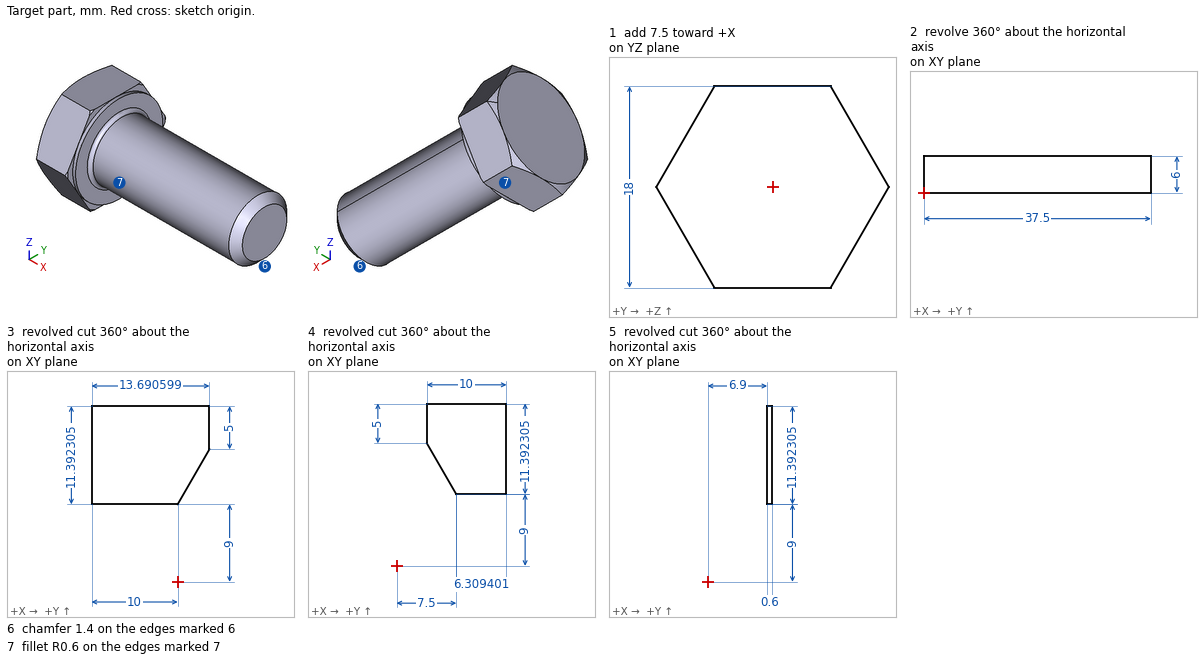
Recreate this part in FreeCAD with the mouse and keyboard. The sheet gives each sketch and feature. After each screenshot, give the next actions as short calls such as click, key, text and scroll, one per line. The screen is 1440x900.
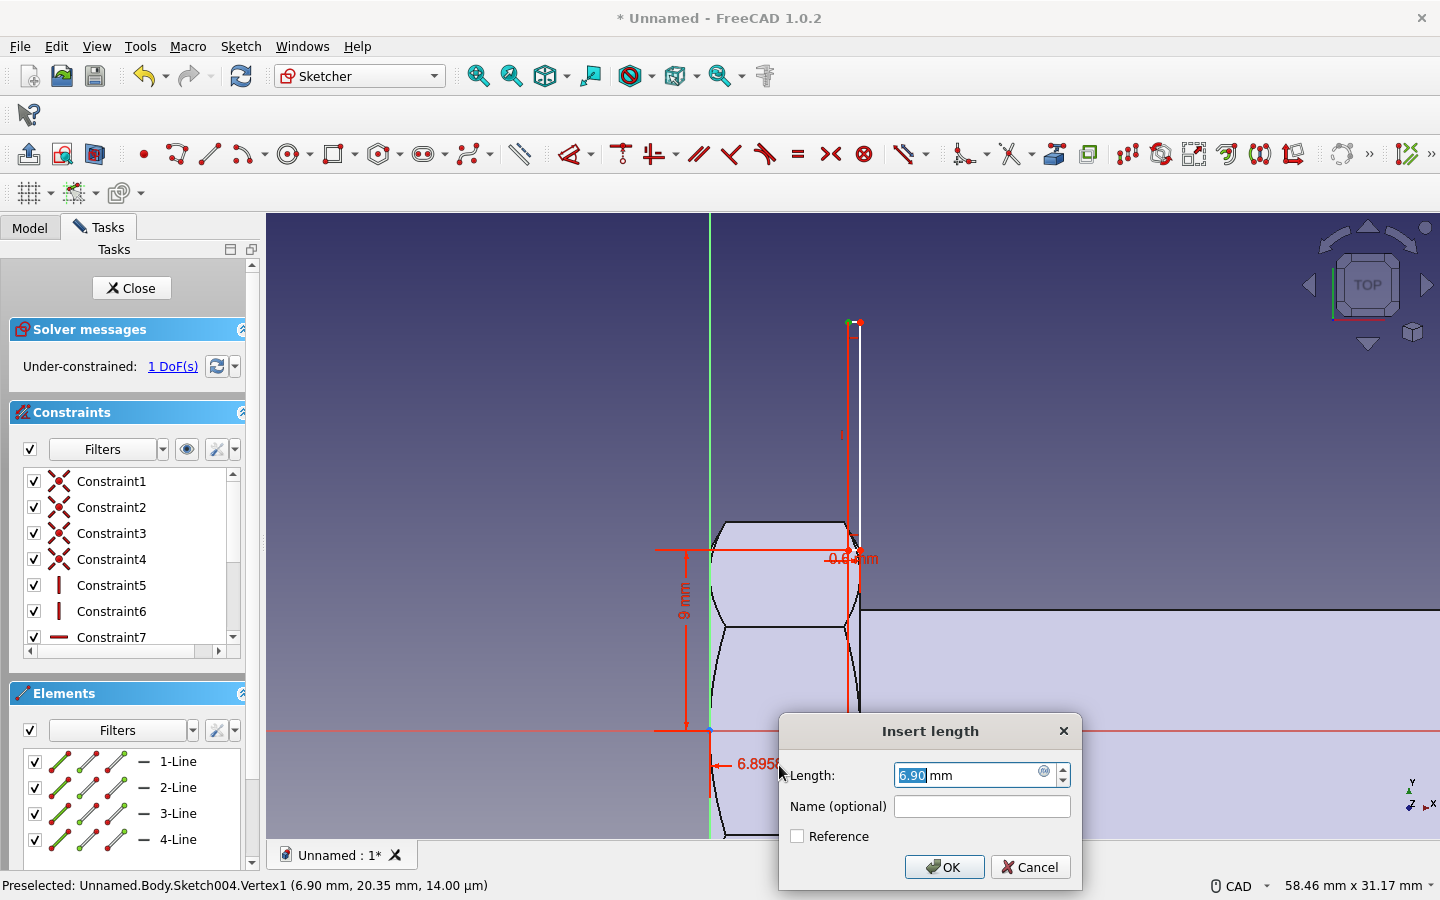
text(6.9)
key(Return)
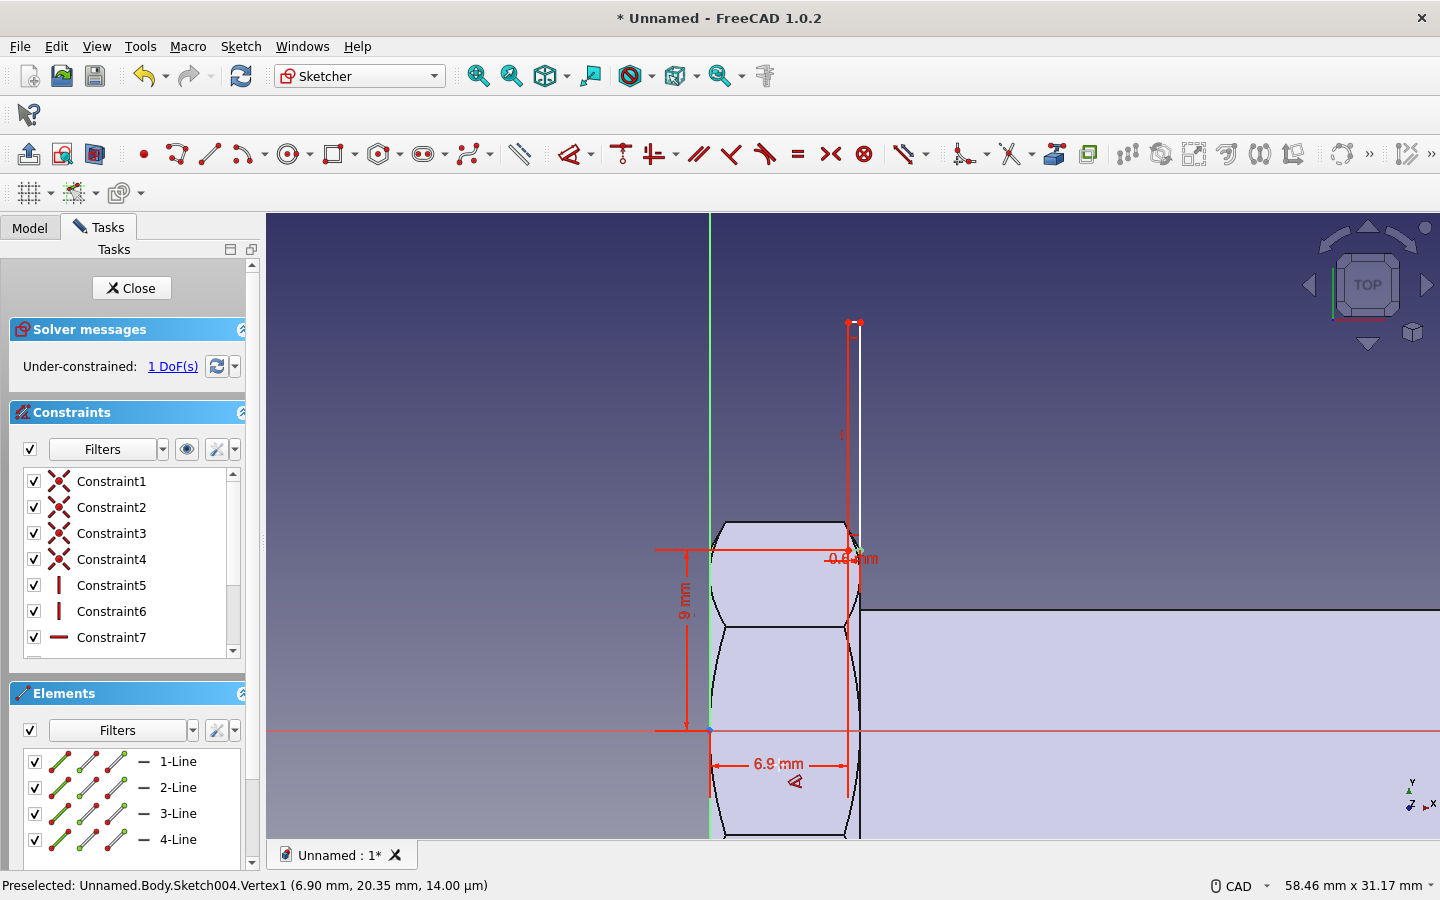
click(848, 391)
click(882, 436)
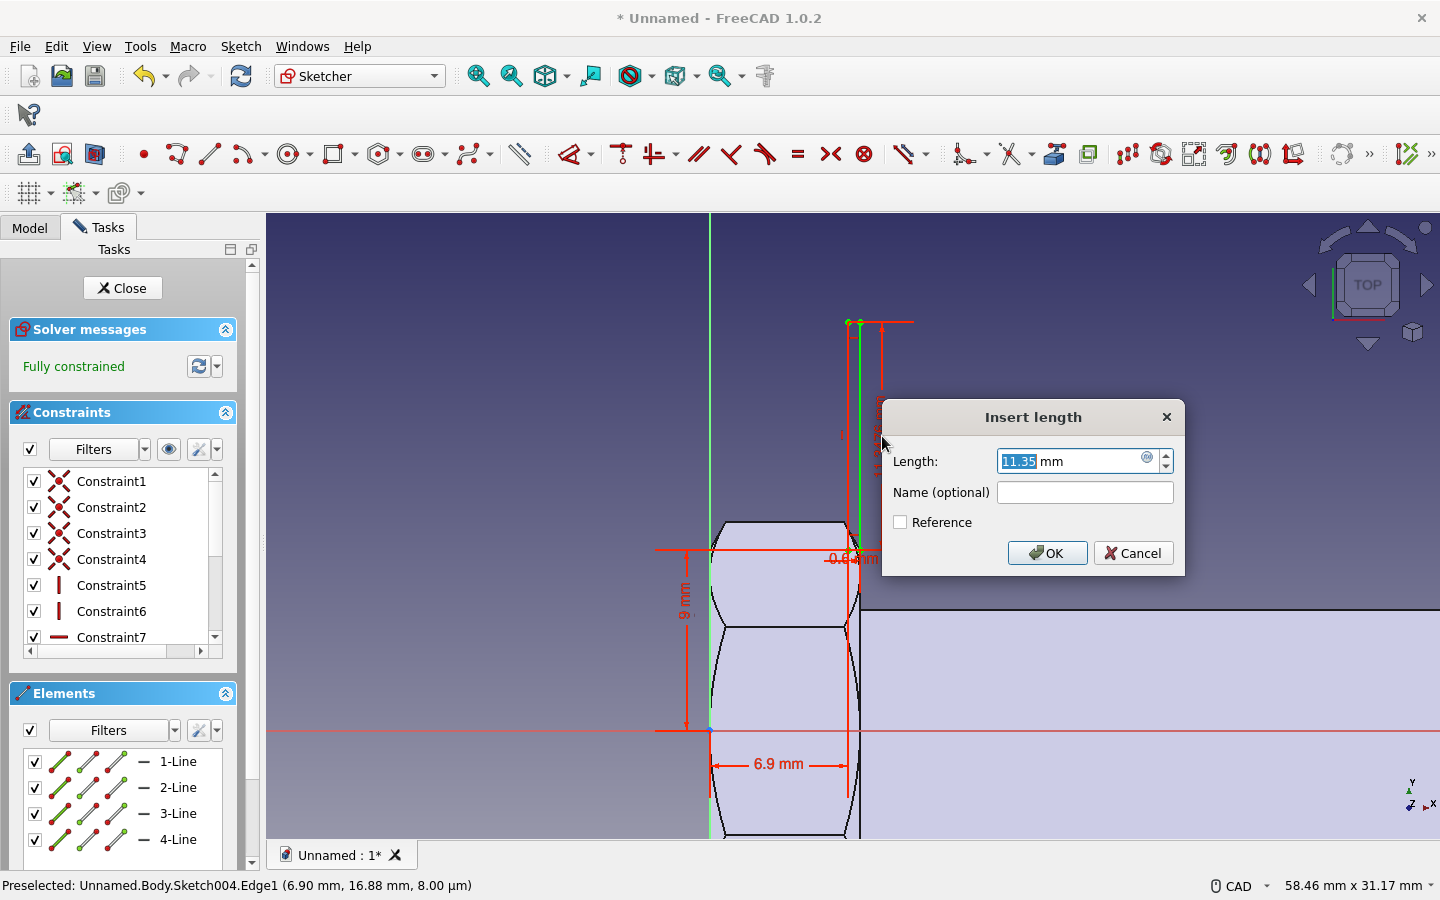
text(11.392305)
key(Return)
key(Escape)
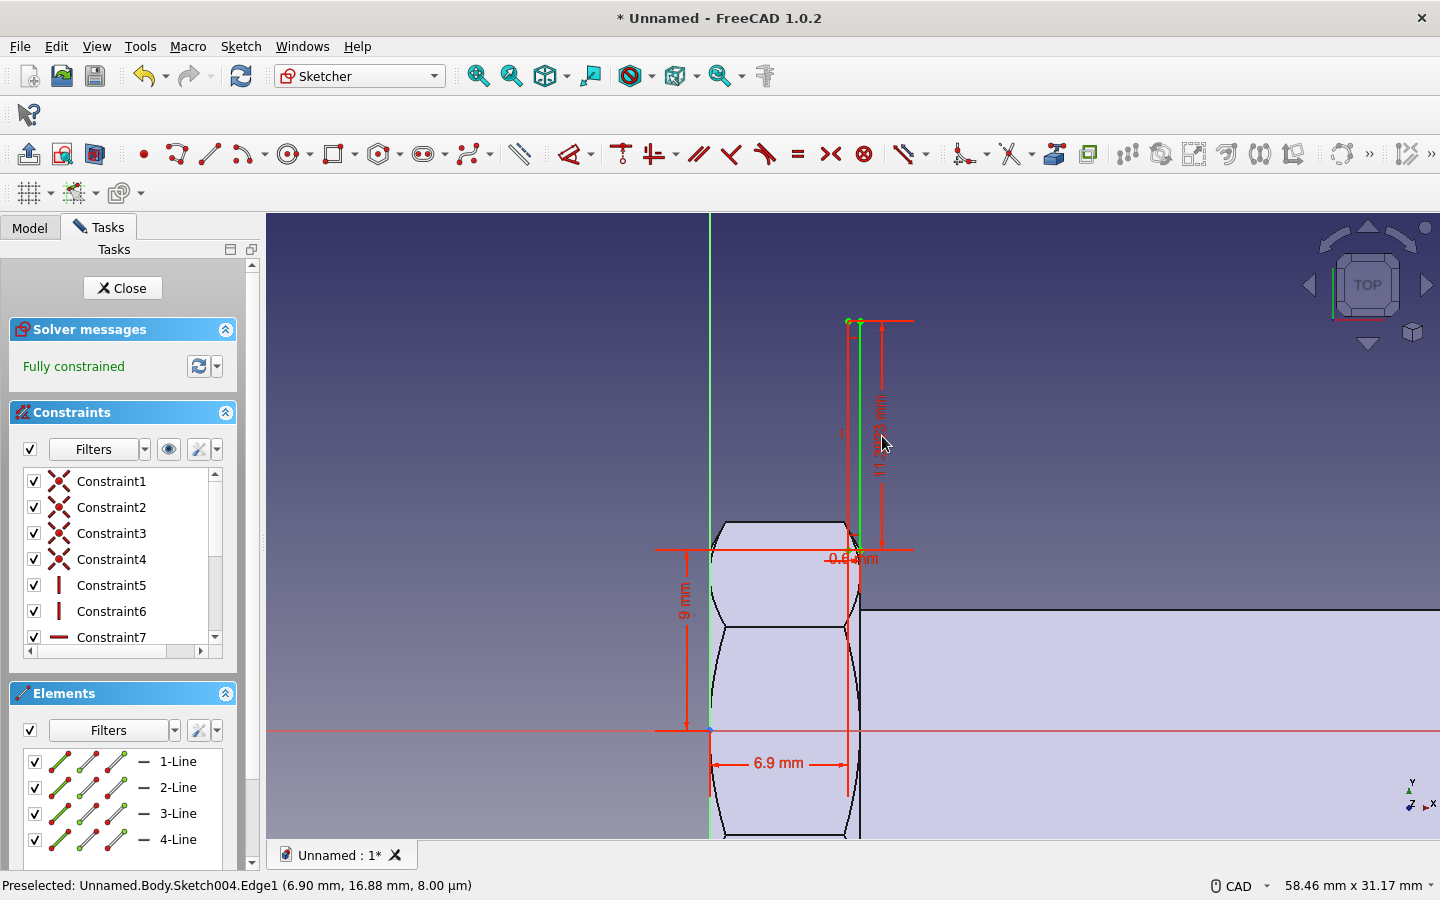
click(123, 288)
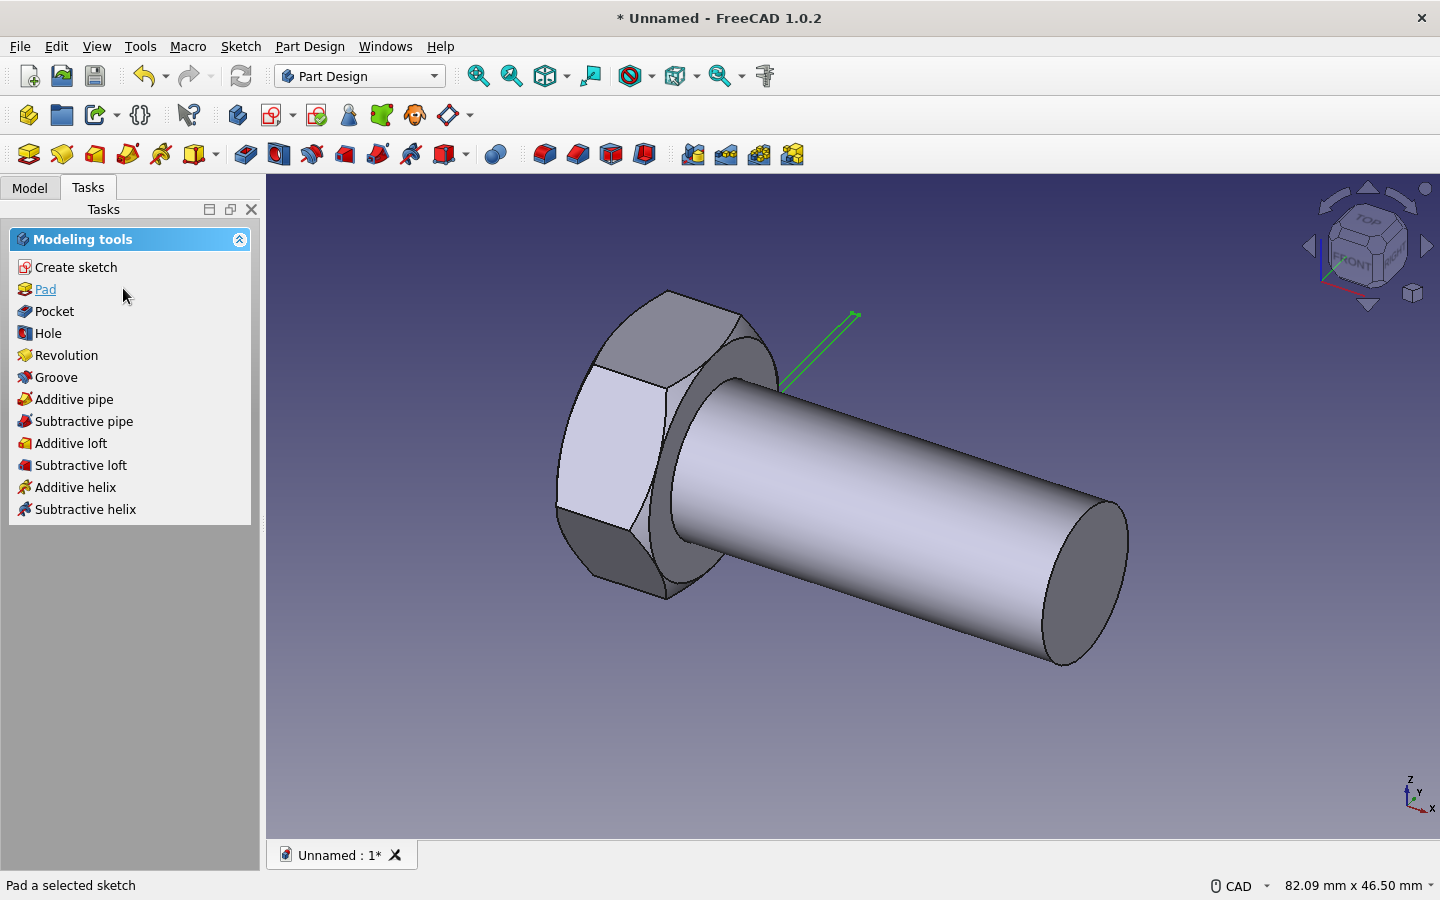
click(312, 154)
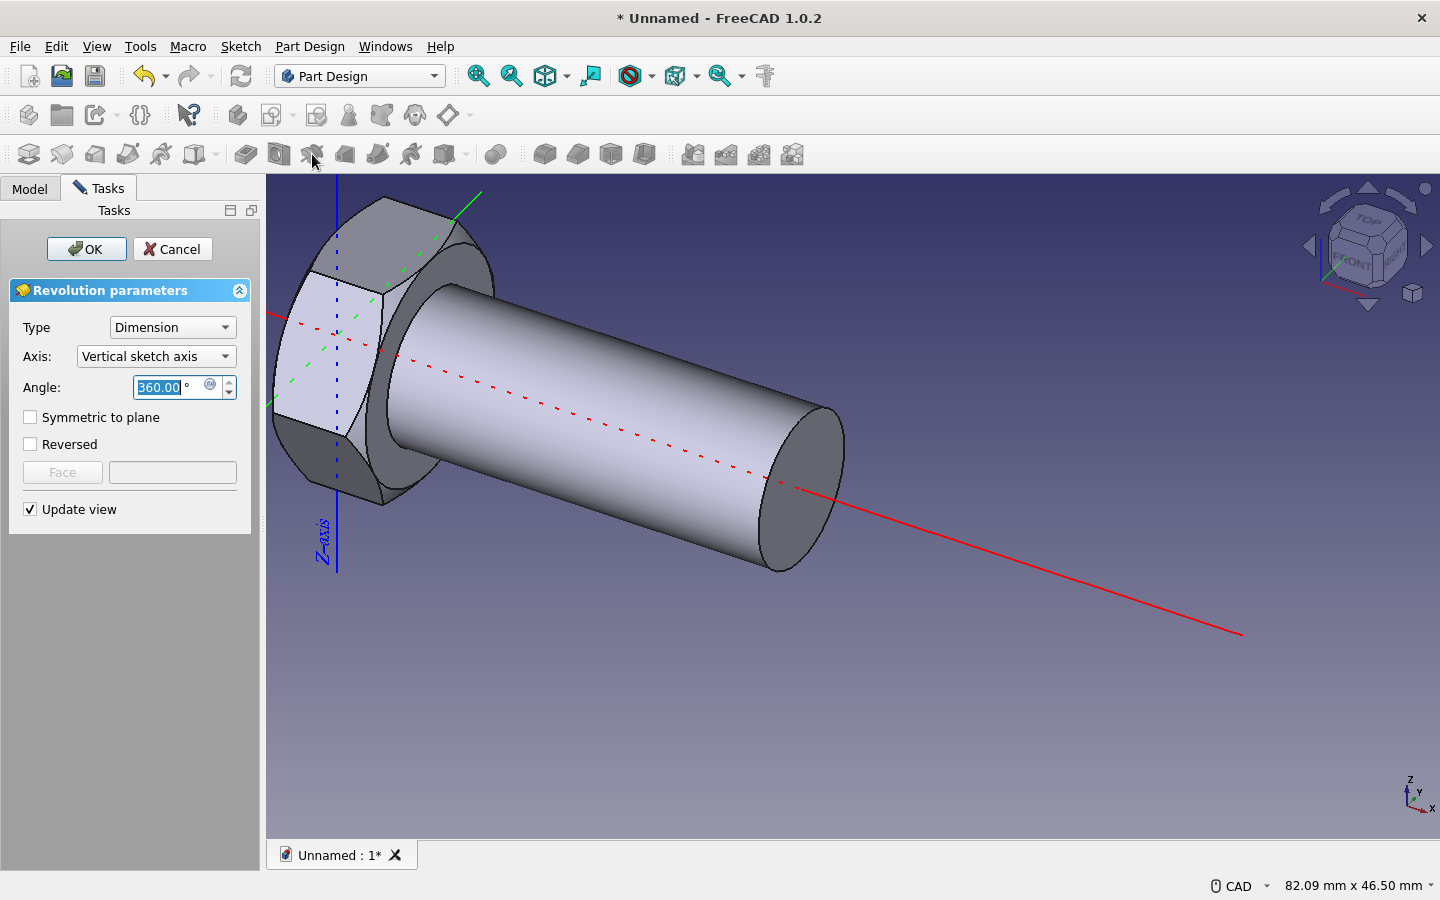
click(157, 356)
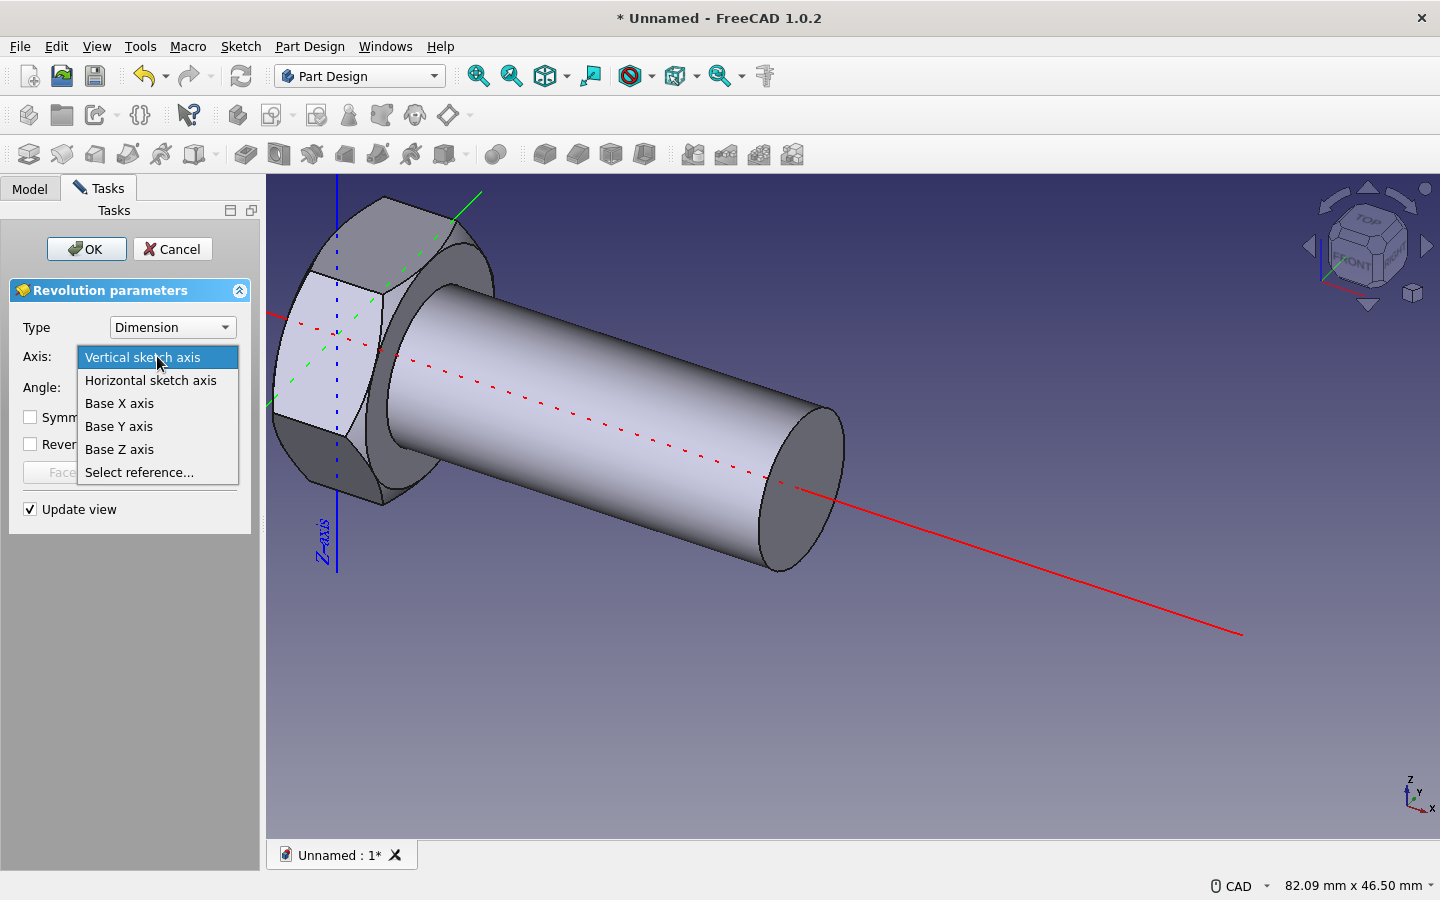
click(156, 380)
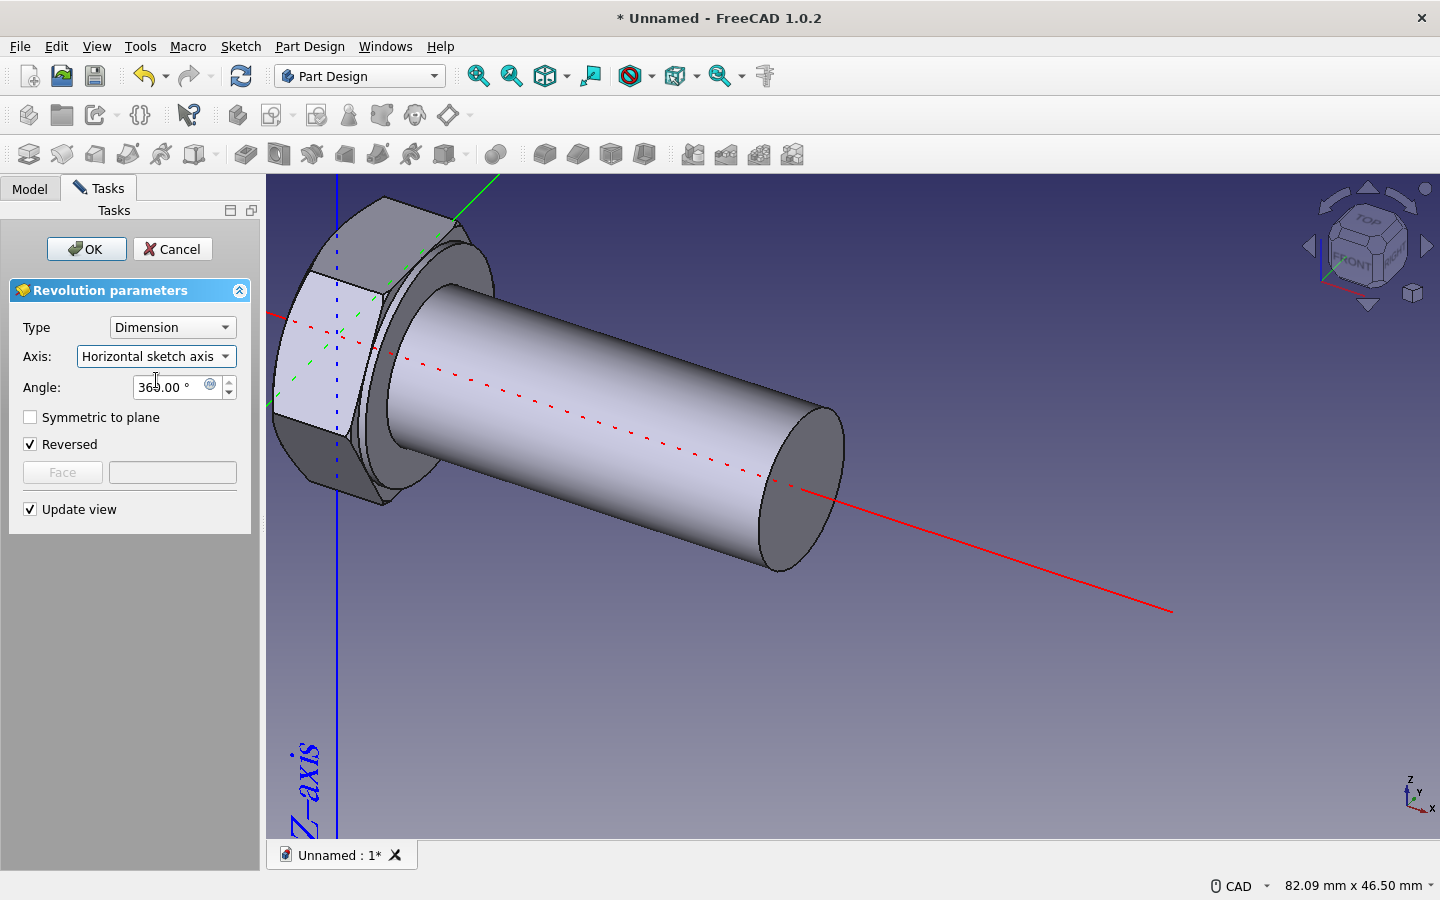
click(87, 249)